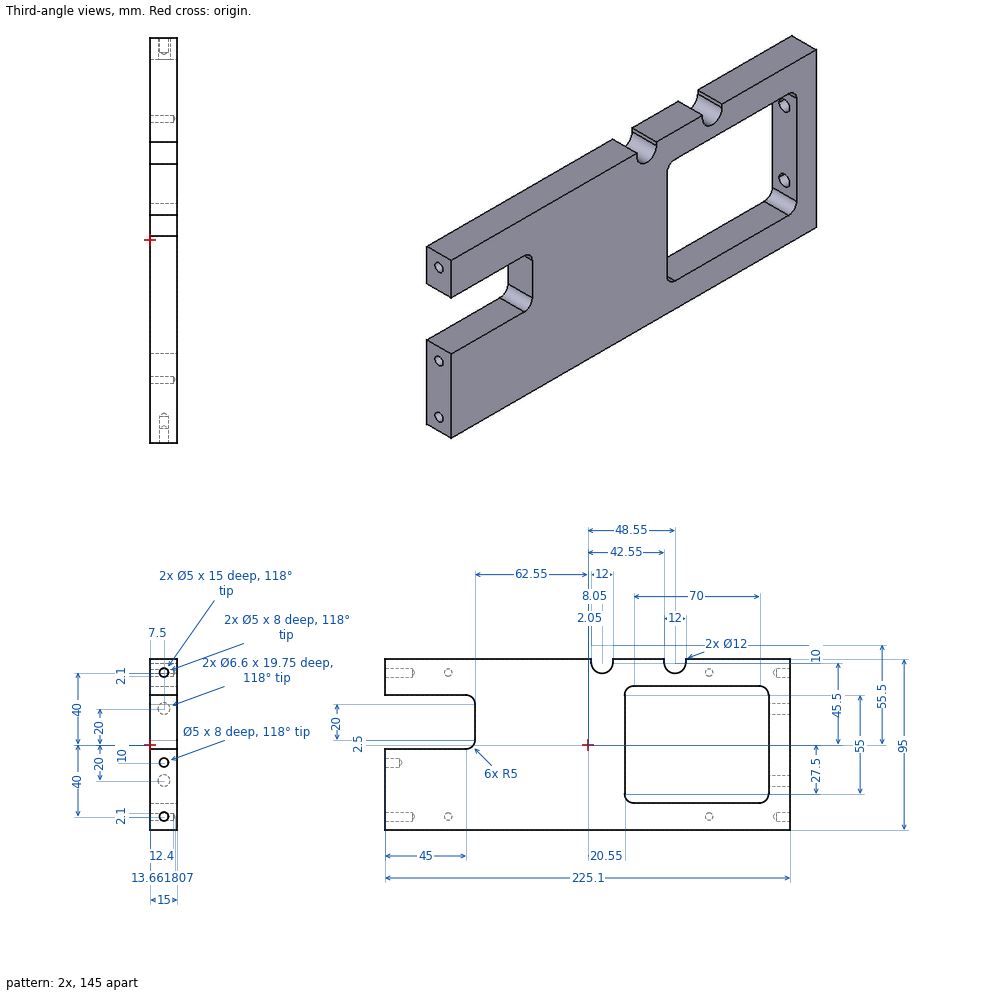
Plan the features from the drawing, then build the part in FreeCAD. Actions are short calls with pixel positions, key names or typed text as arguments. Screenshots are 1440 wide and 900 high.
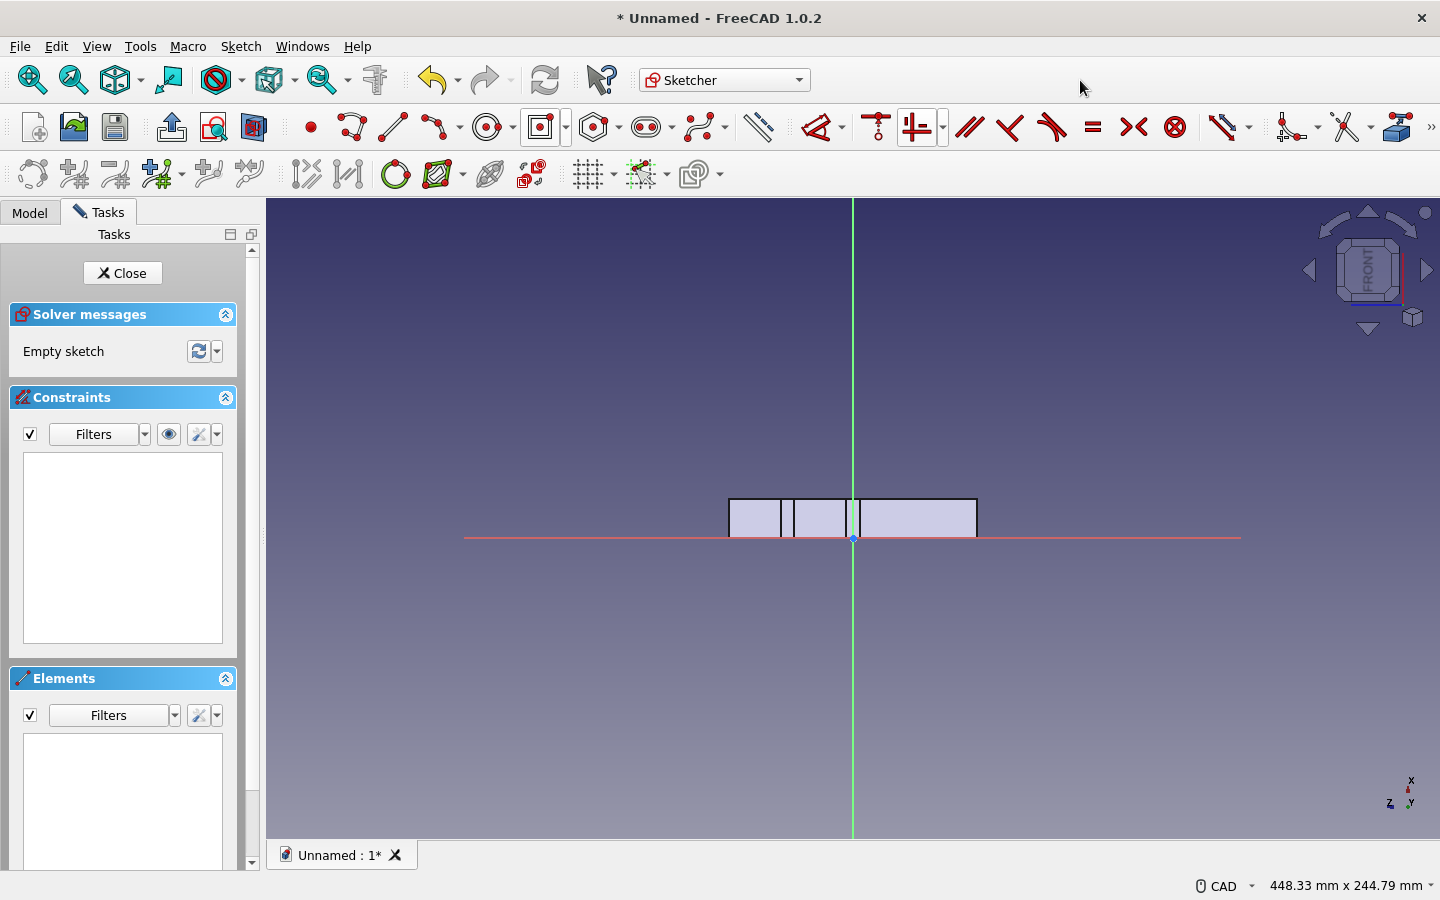
scroll(883, 528, up, 6)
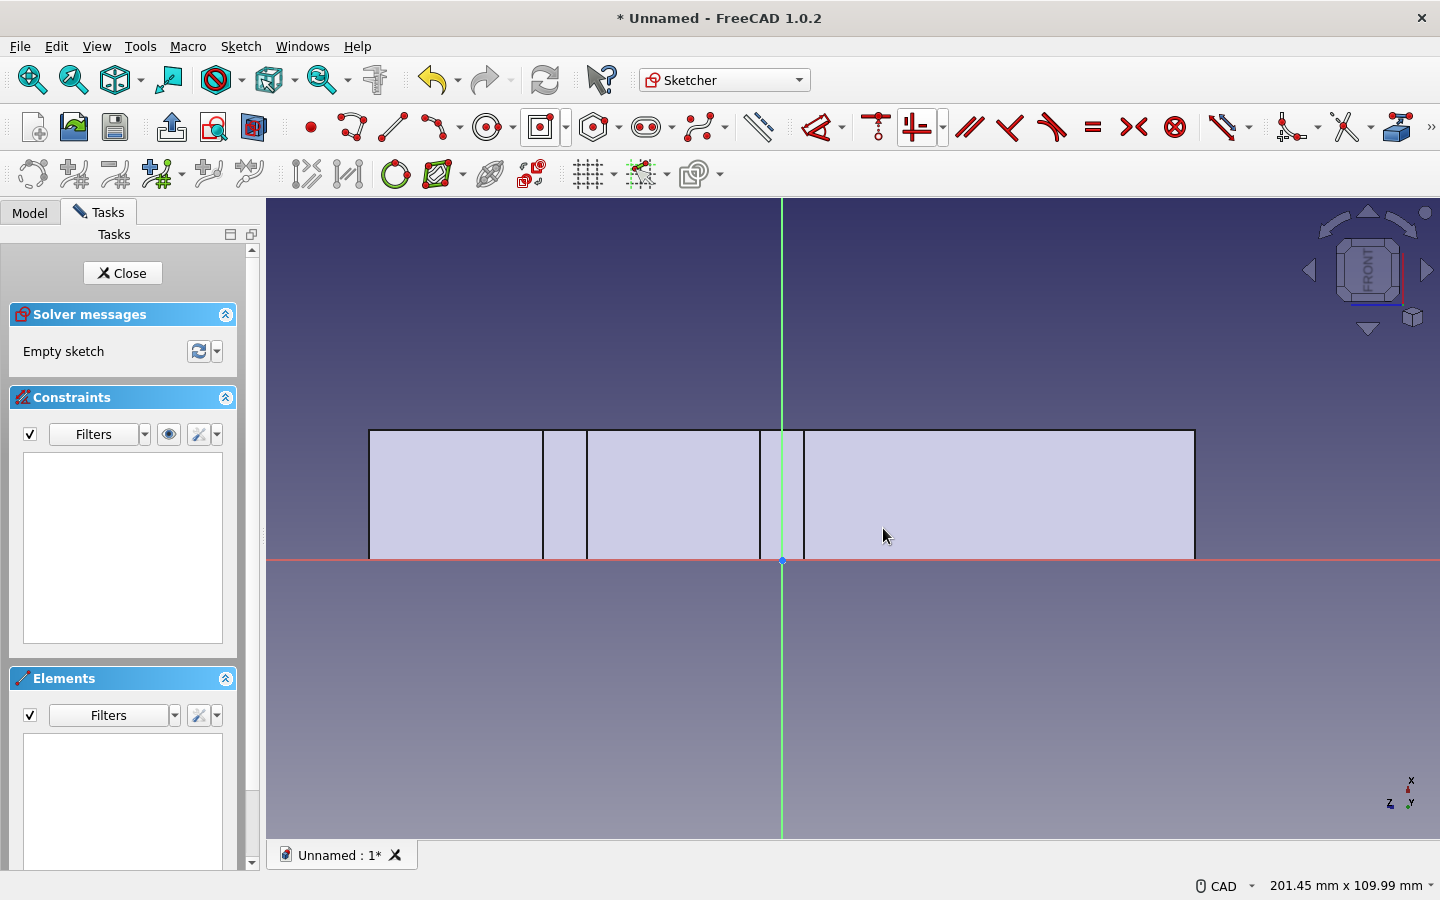
click(486, 128)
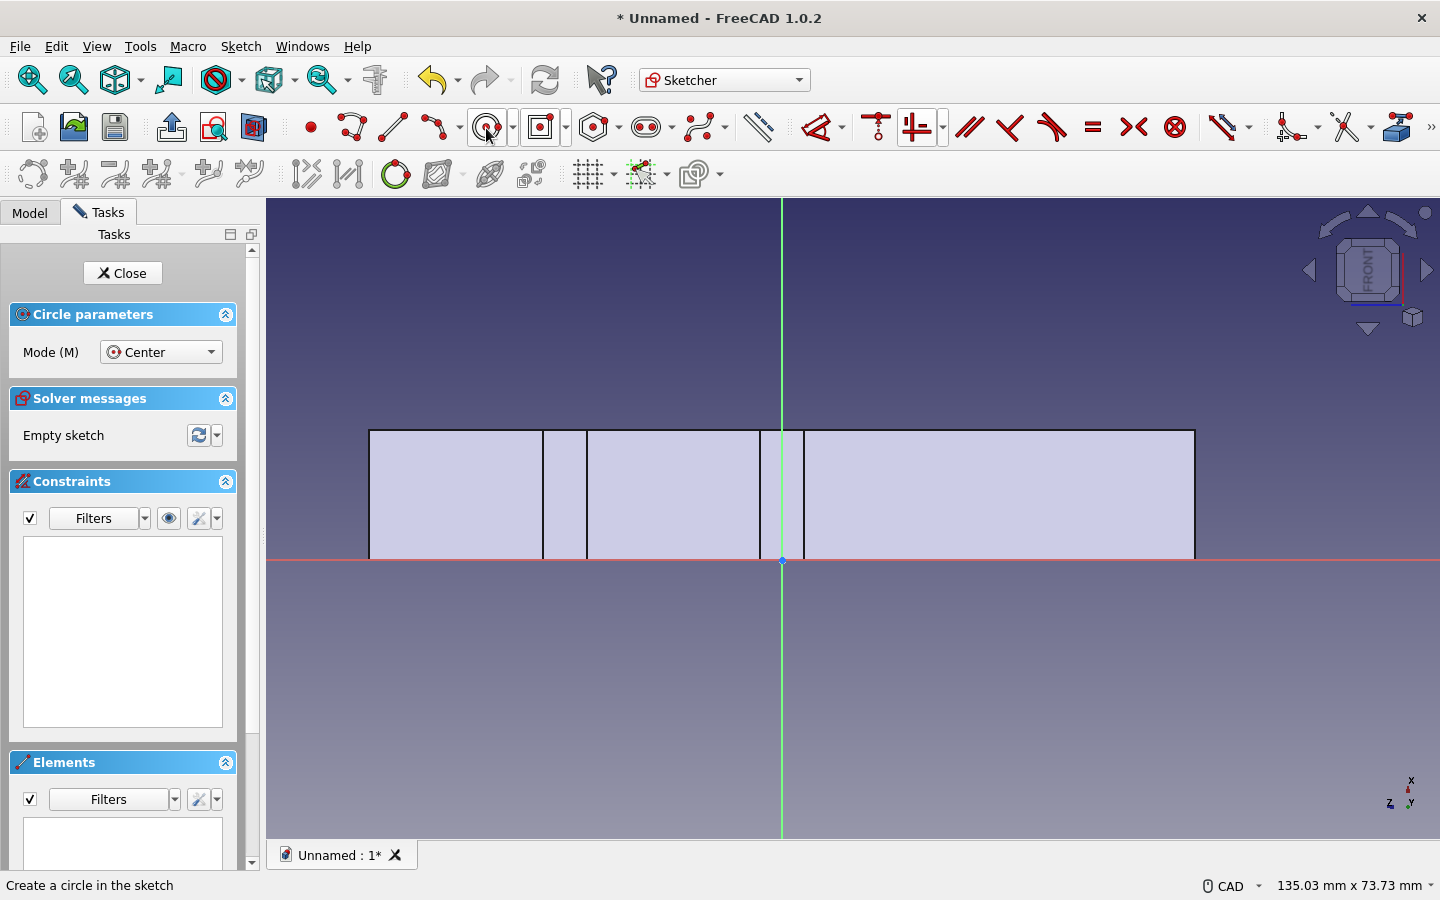
click(434, 495)
move(450, 480)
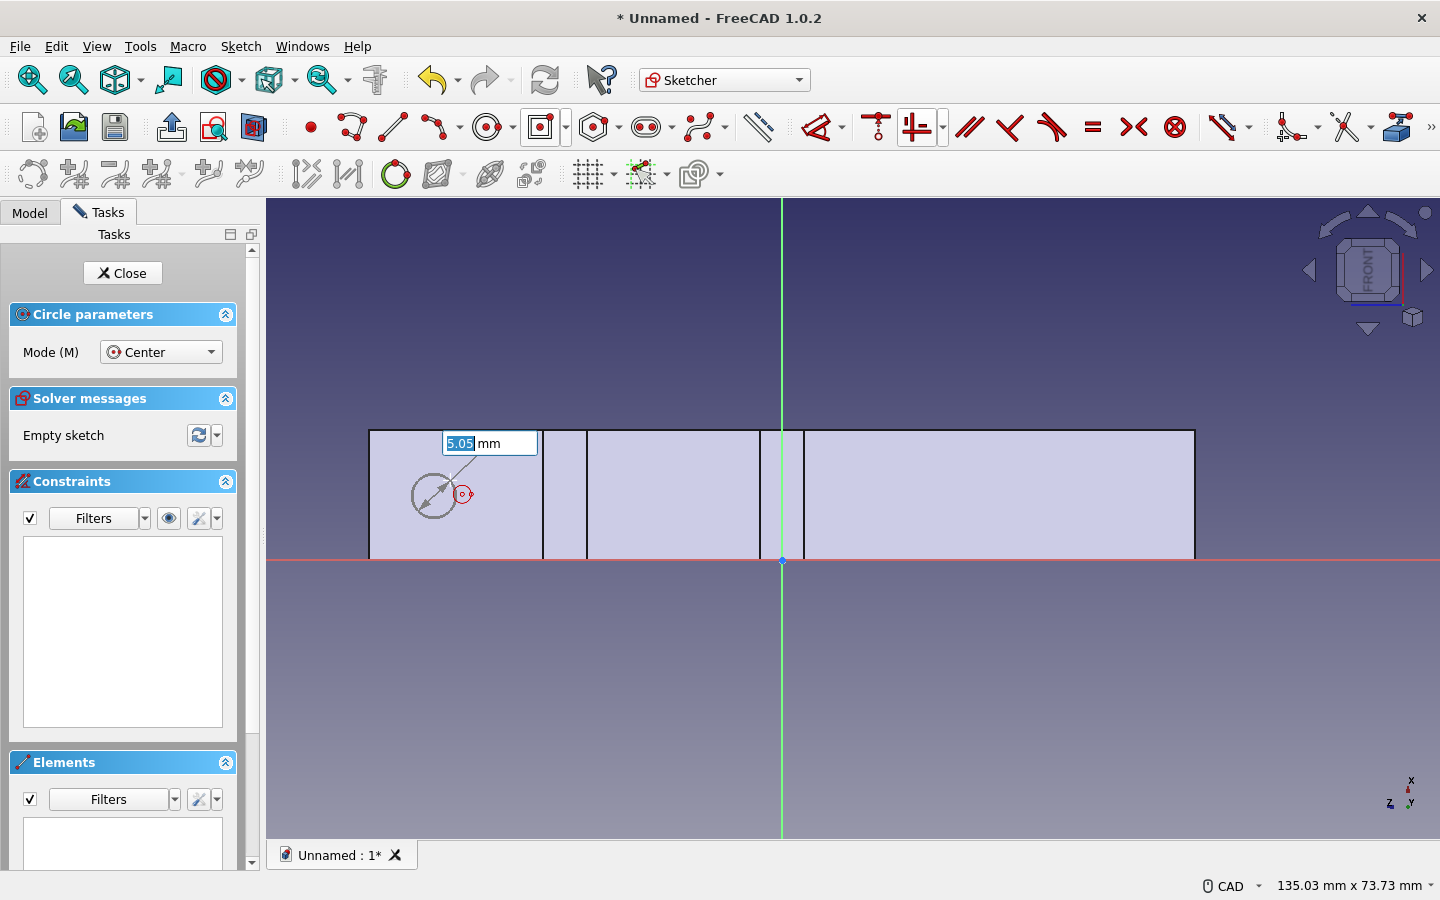
text(5)
key(Return)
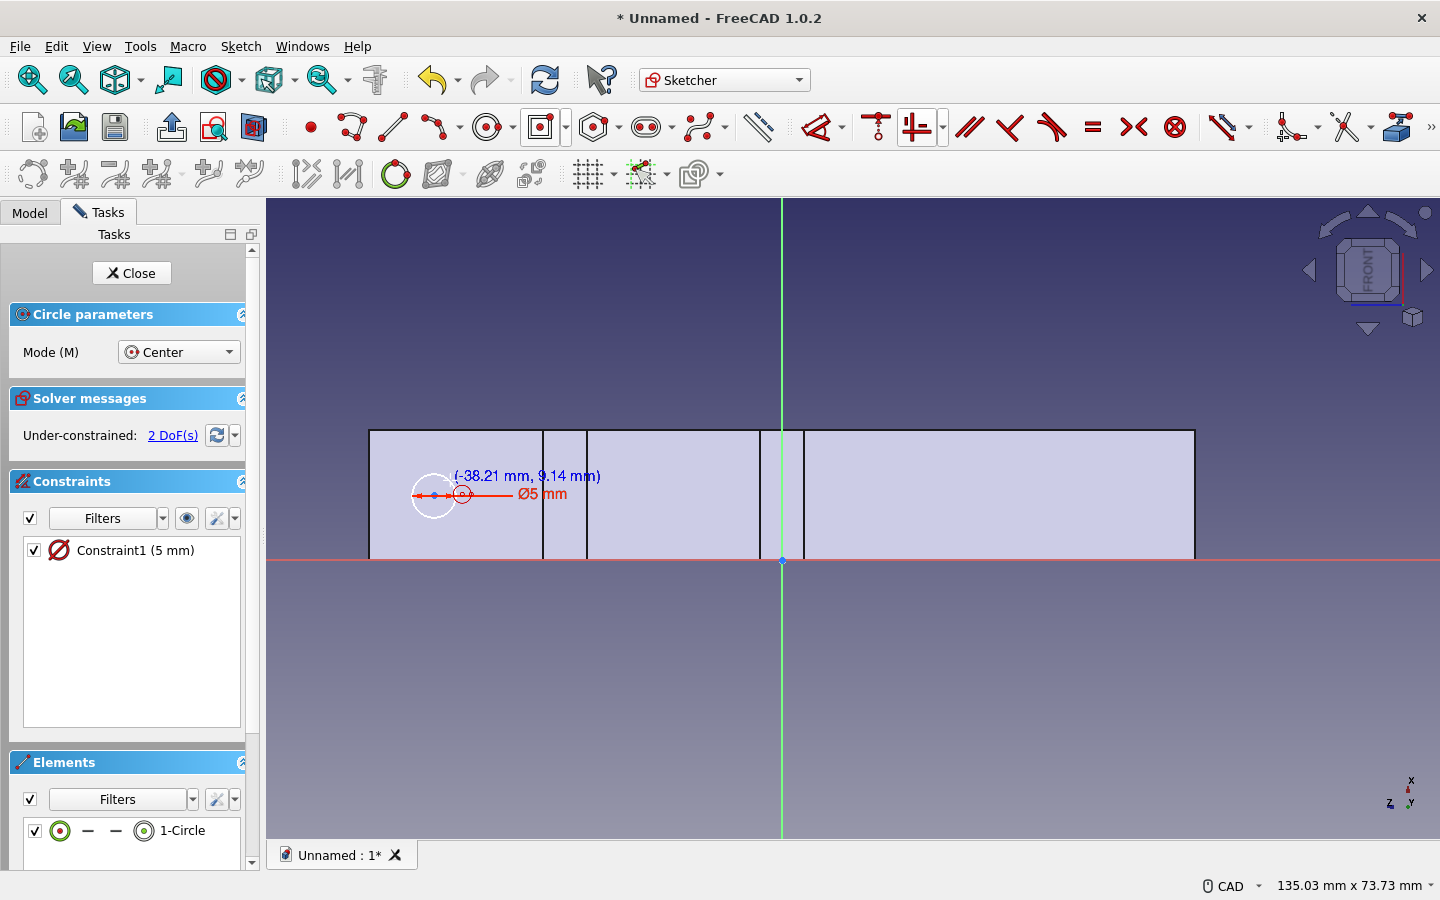
click(1130, 495)
move(1145, 480)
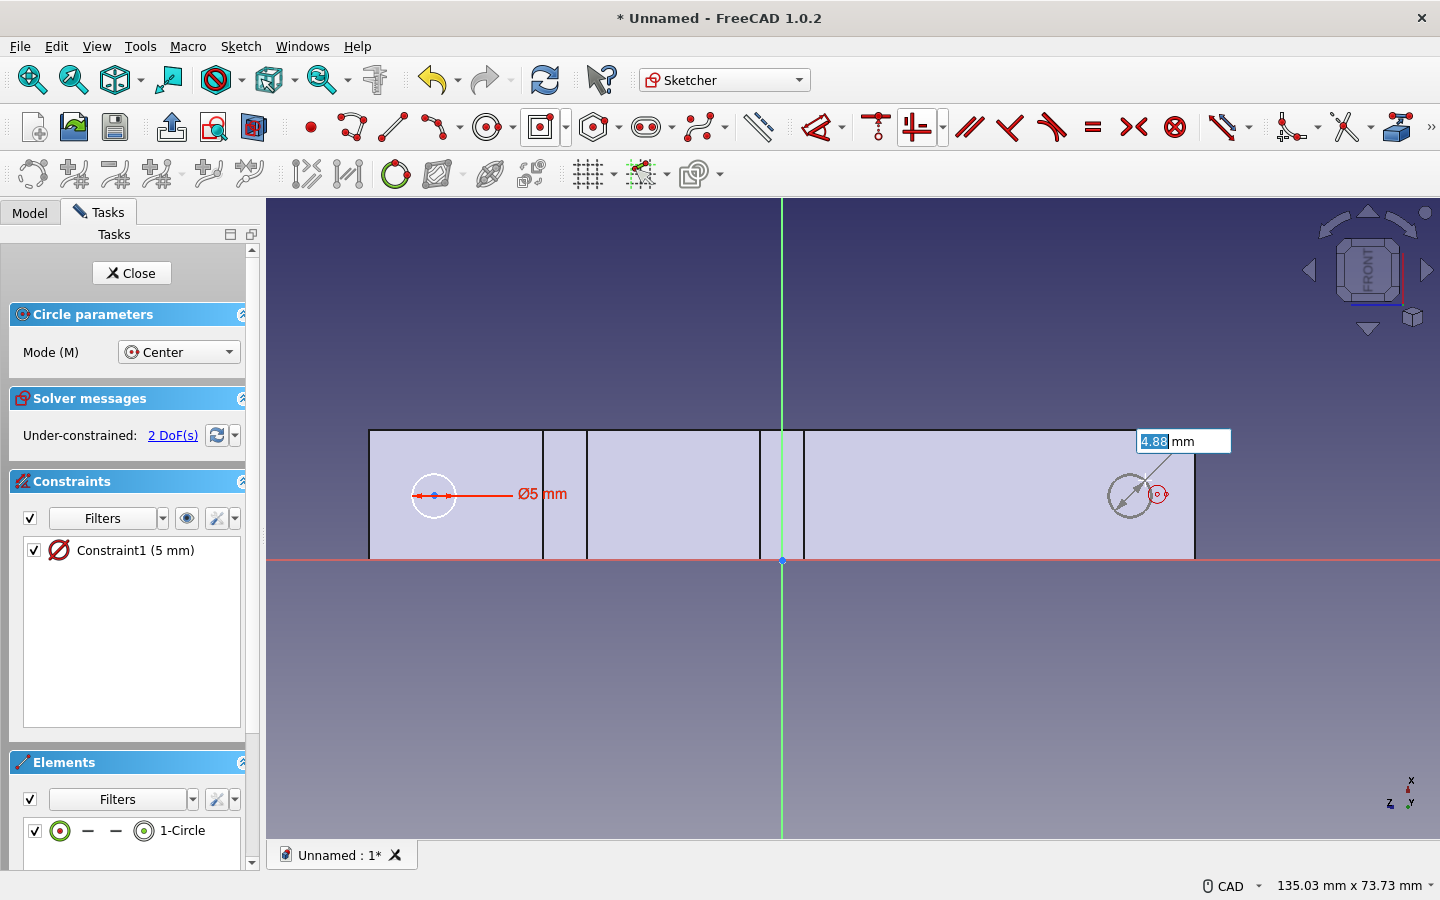
text(5)
key(Return)
key(Escape)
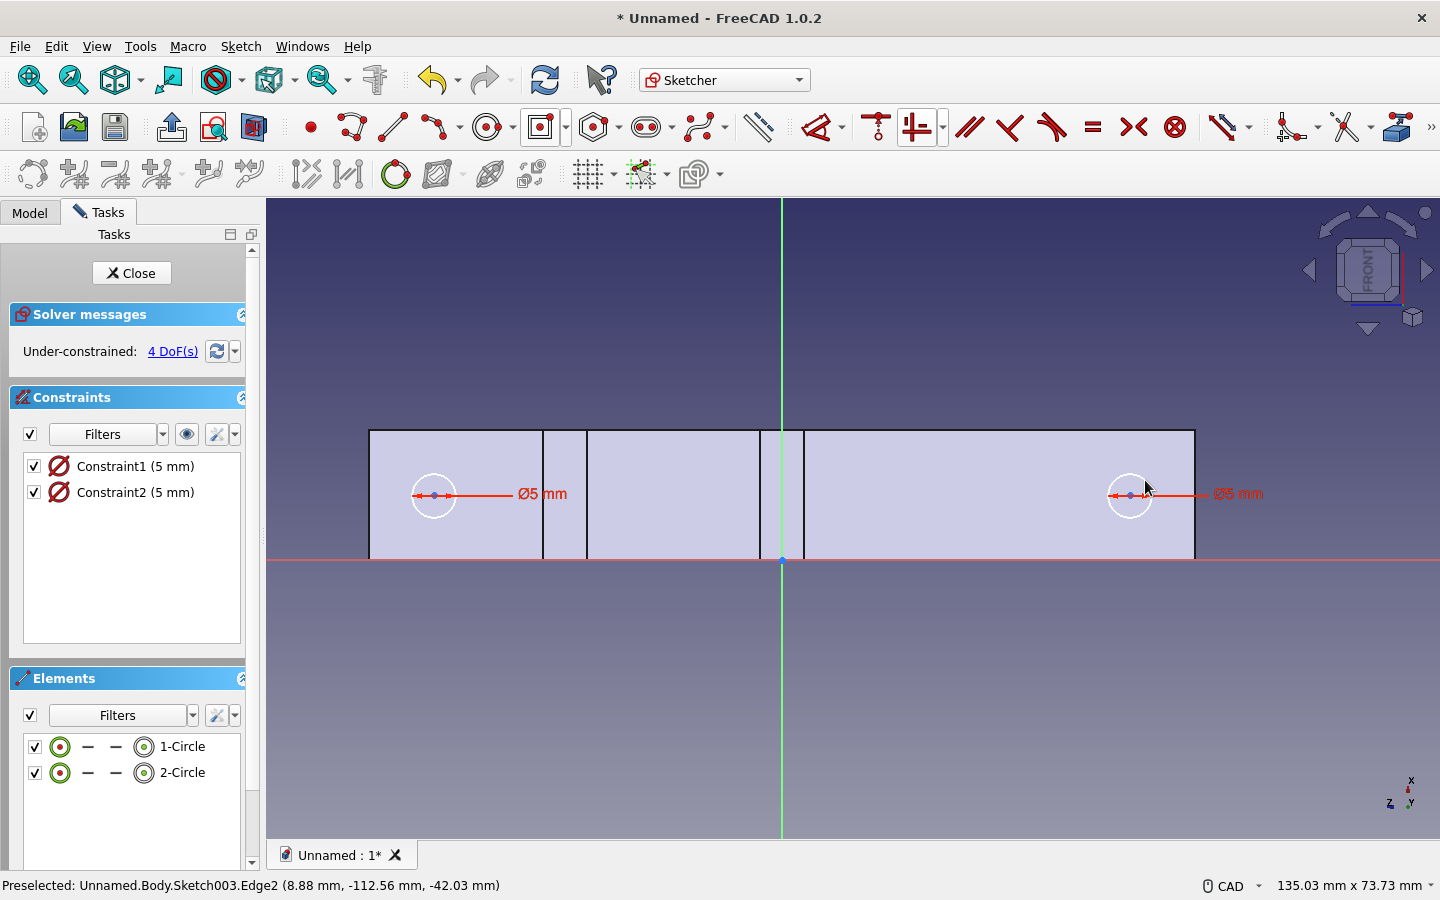
click(434, 496)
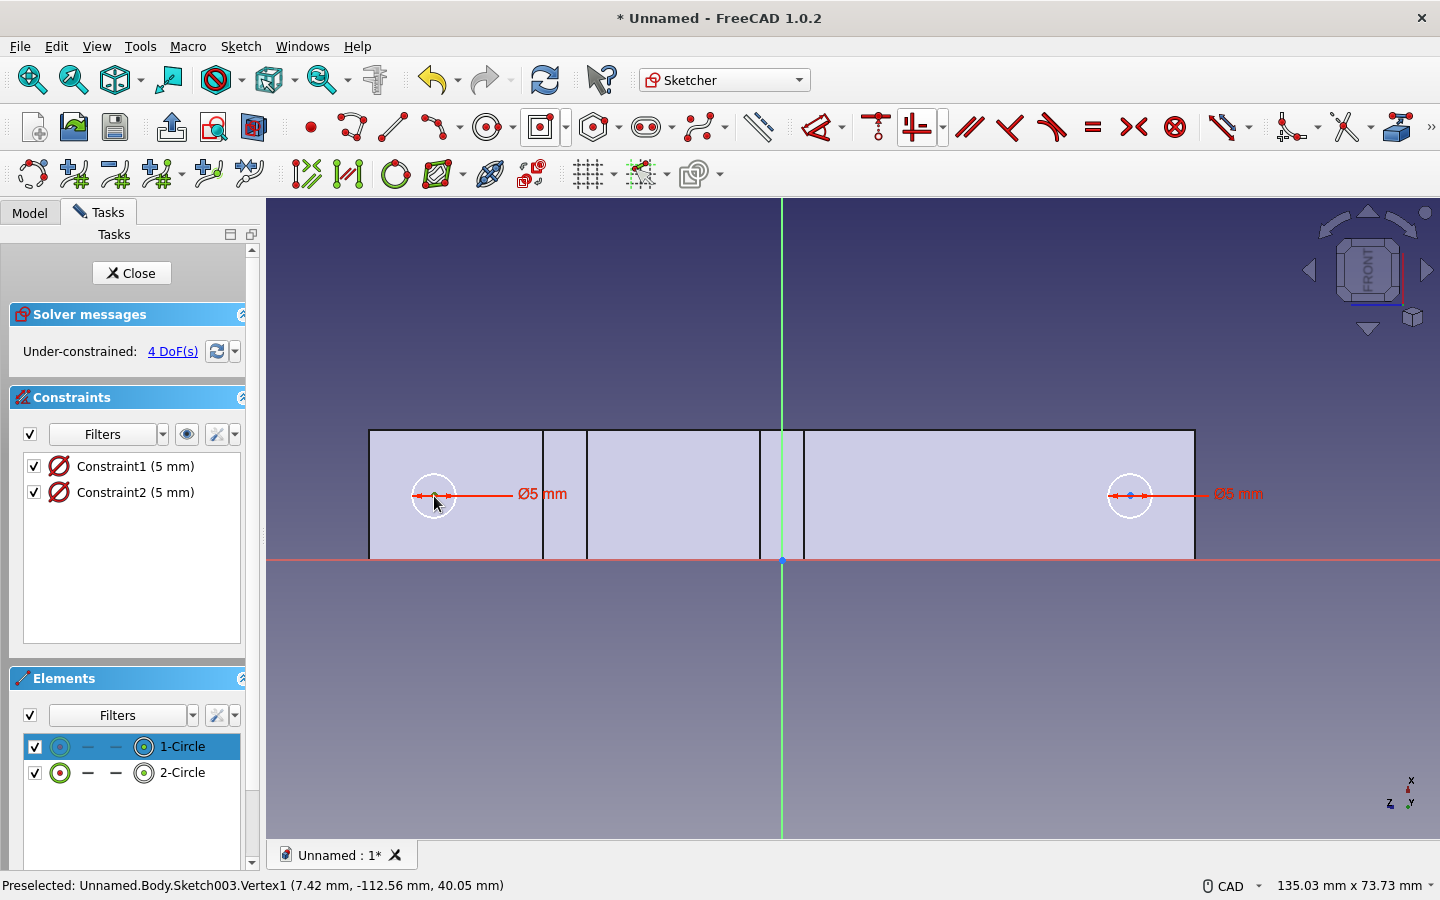
click(1130, 496)